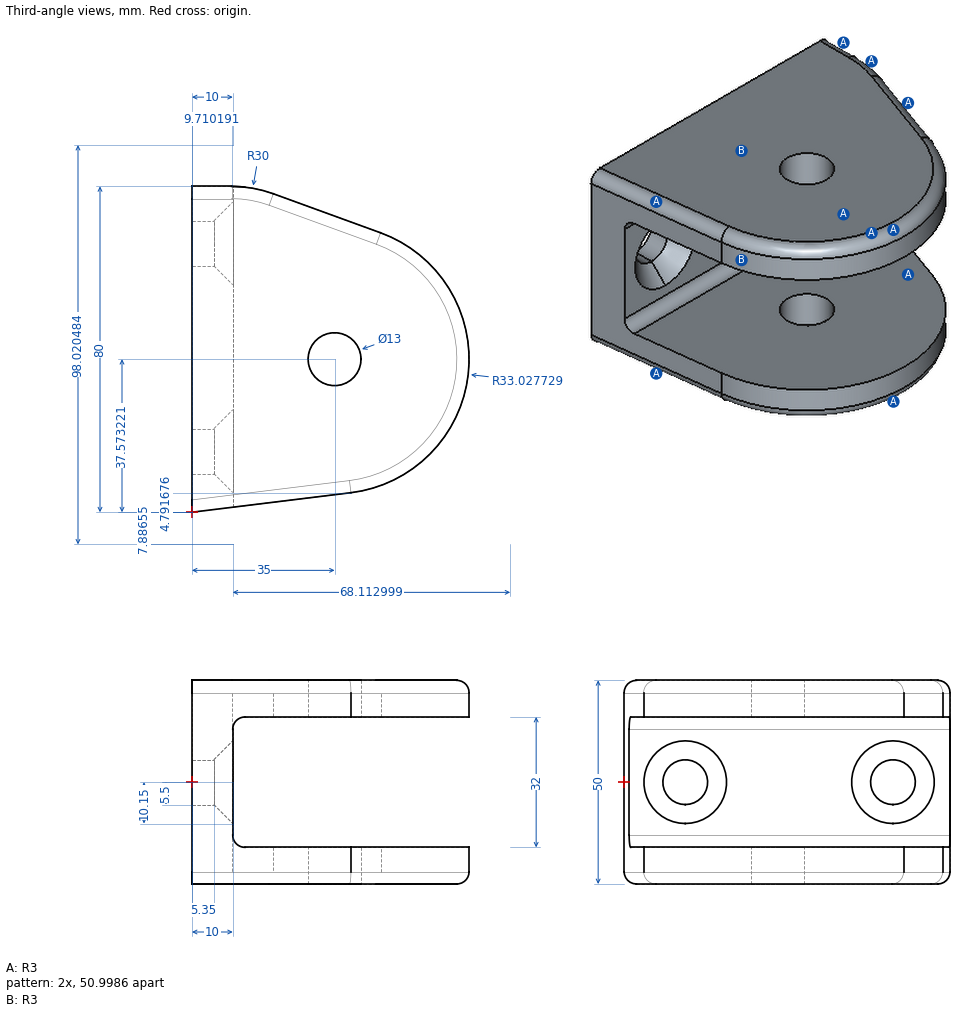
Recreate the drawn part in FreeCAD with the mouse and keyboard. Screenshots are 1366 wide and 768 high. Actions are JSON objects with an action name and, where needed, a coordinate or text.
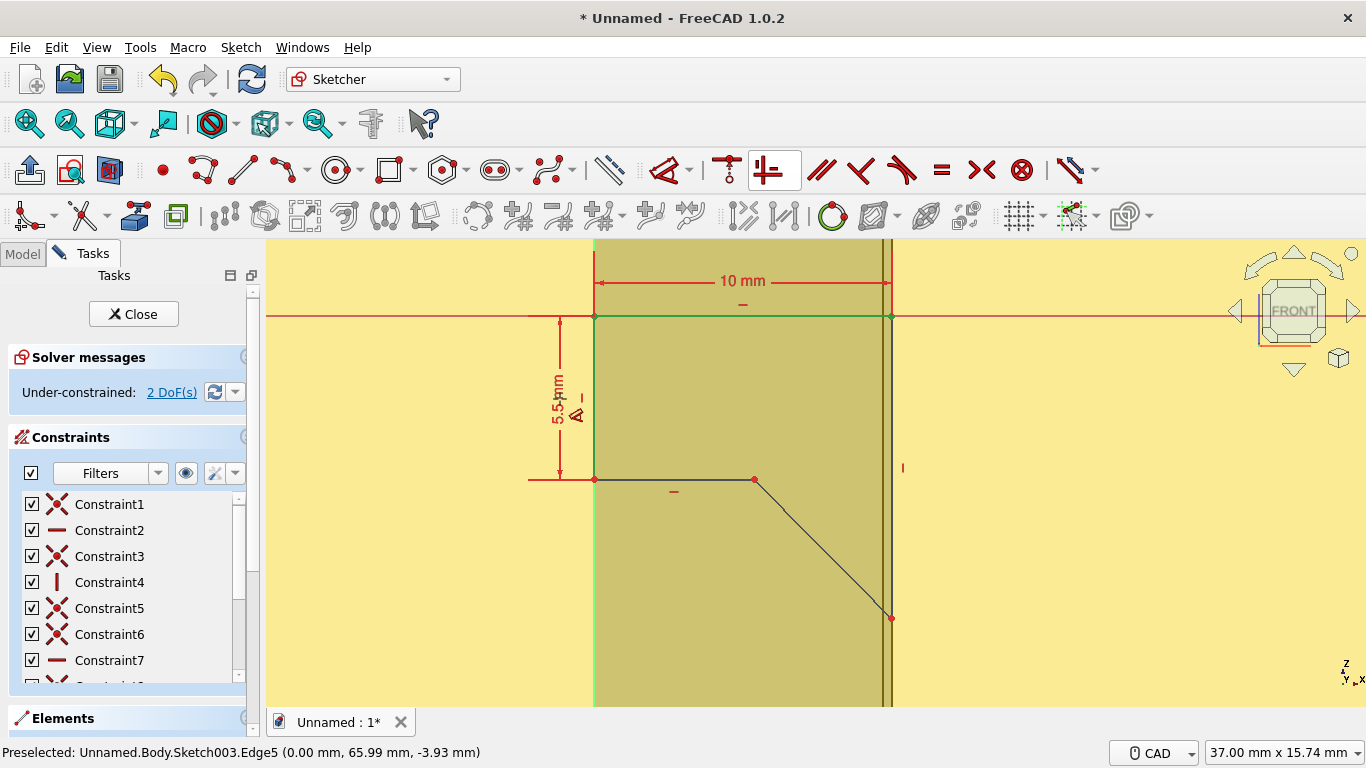
{"action": "left_click", "coordinate": [706, 480]}
{"action": "left_click", "coordinate": [674, 514]}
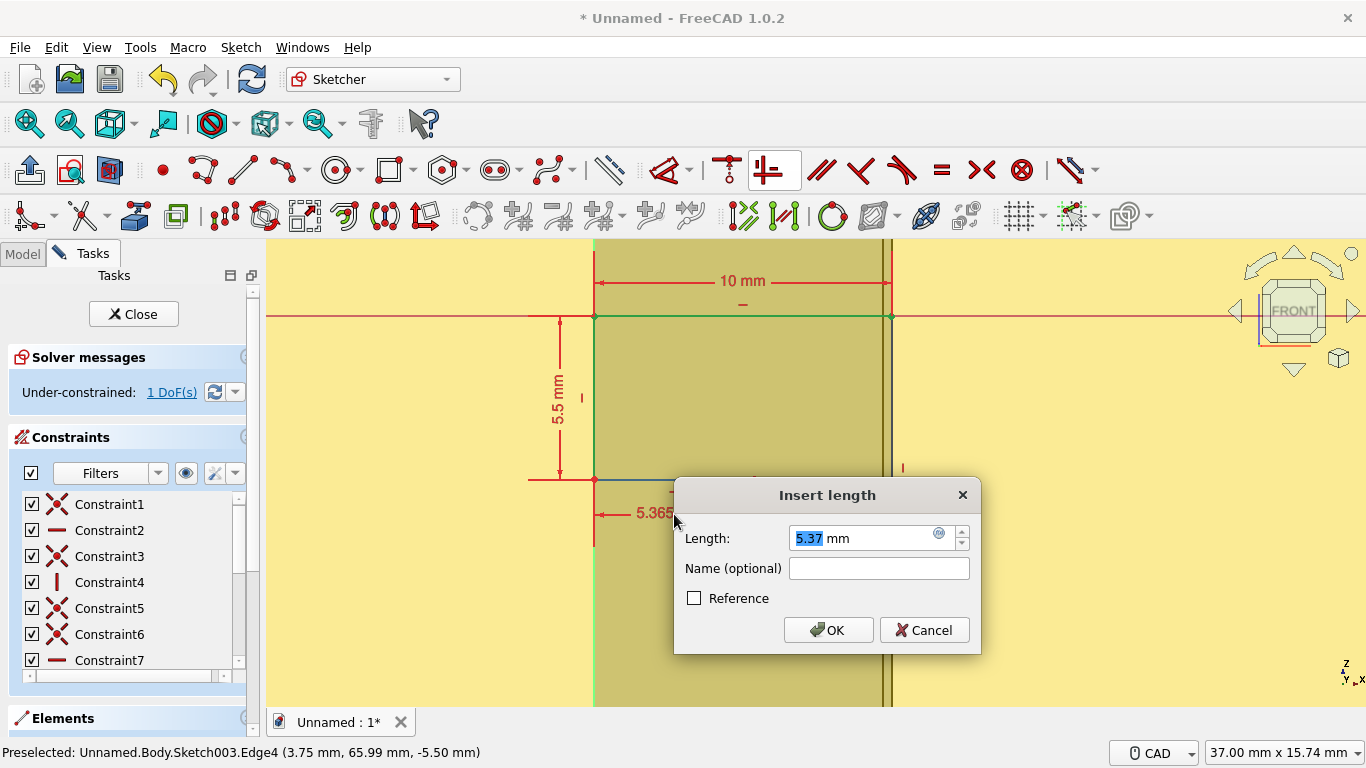
{"action": "type", "text": "5.35"}
{"action": "key", "text": "Return"}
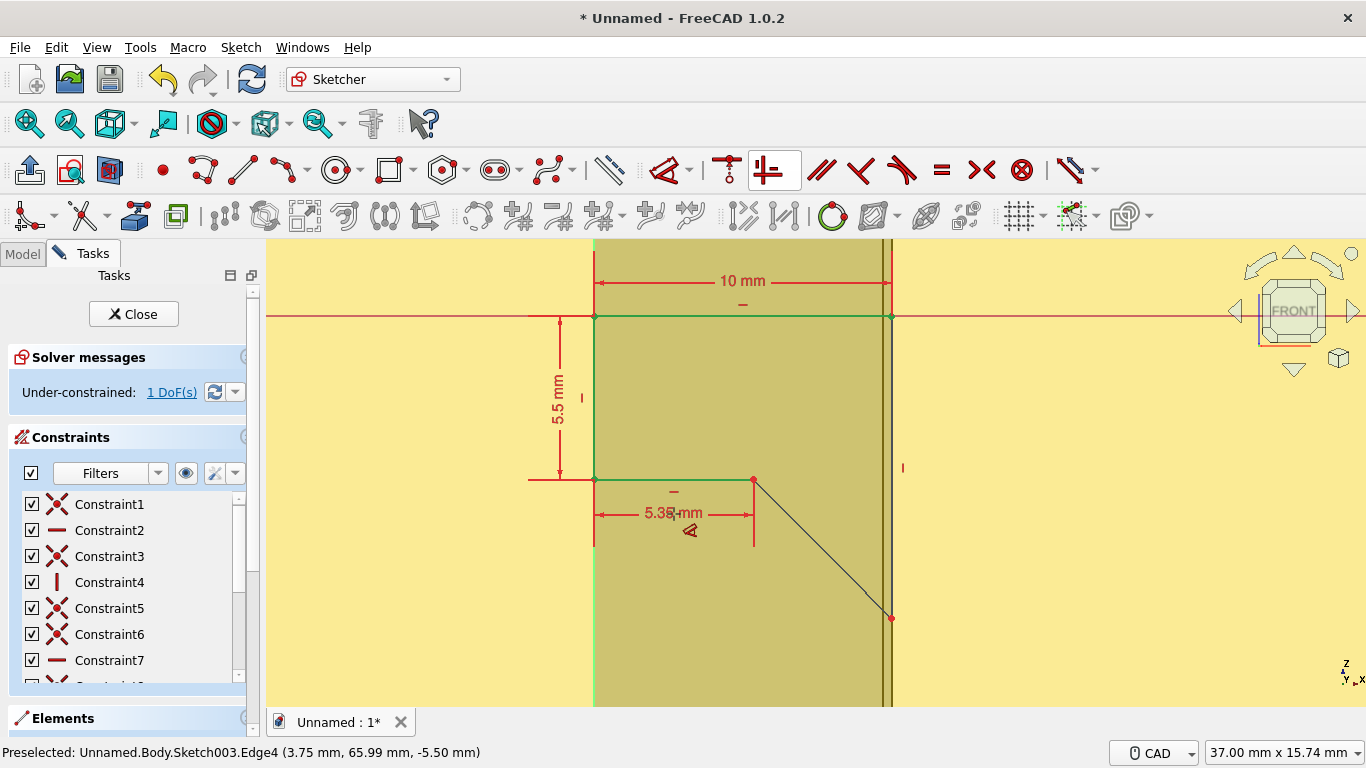
{"action": "left_click", "coordinate": [892, 407]}
{"action": "left_click", "coordinate": [926, 468]}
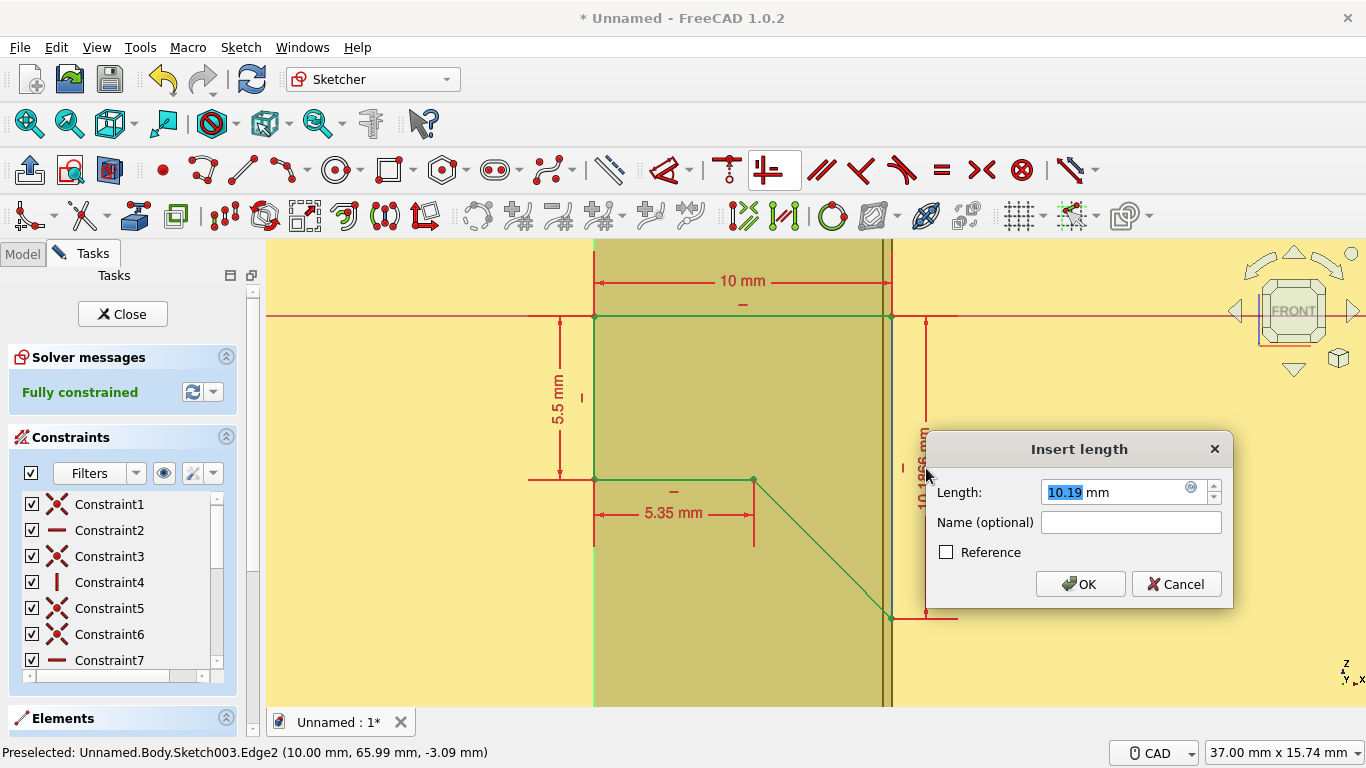
{"action": "type", "text": "10.15"}
{"action": "key", "text": "Return"}
{"action": "key", "text": "Escape"}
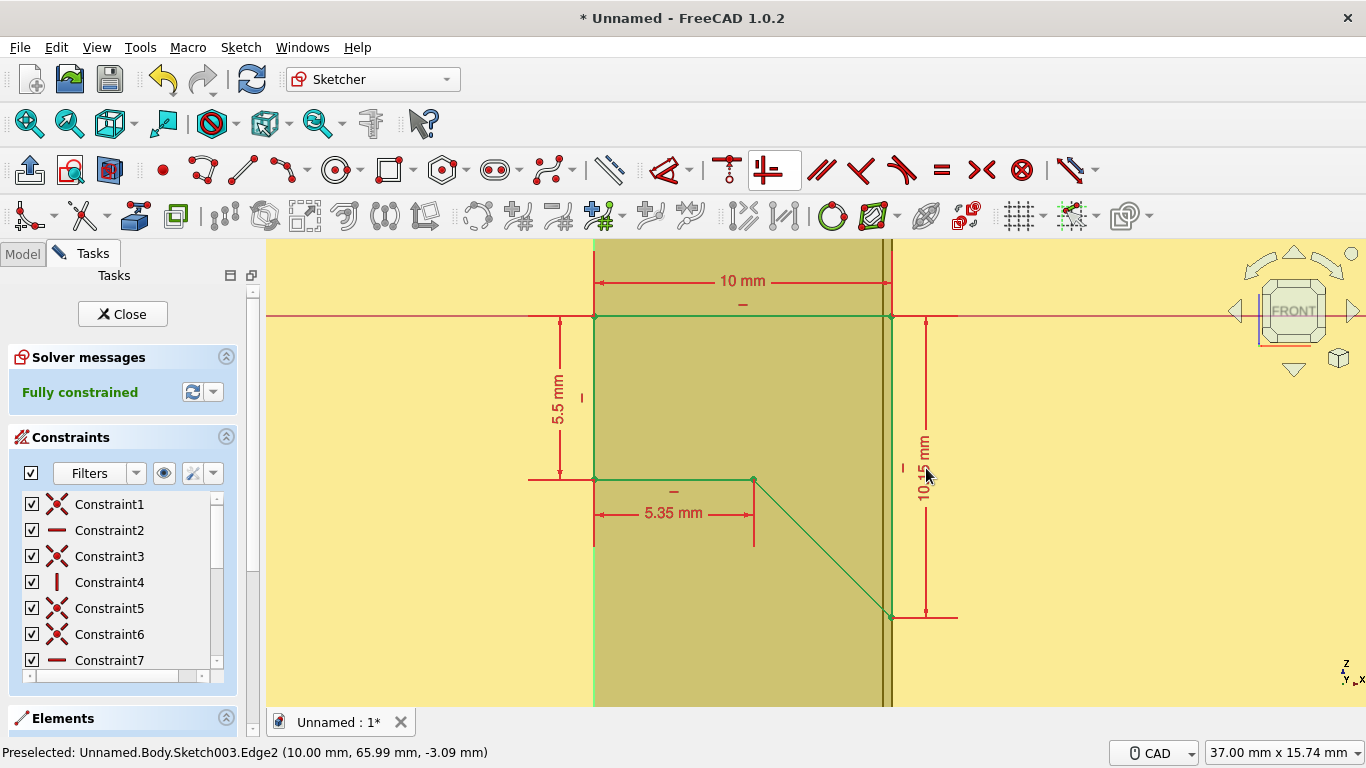
{"action": "left_click", "coordinate": [123, 314]}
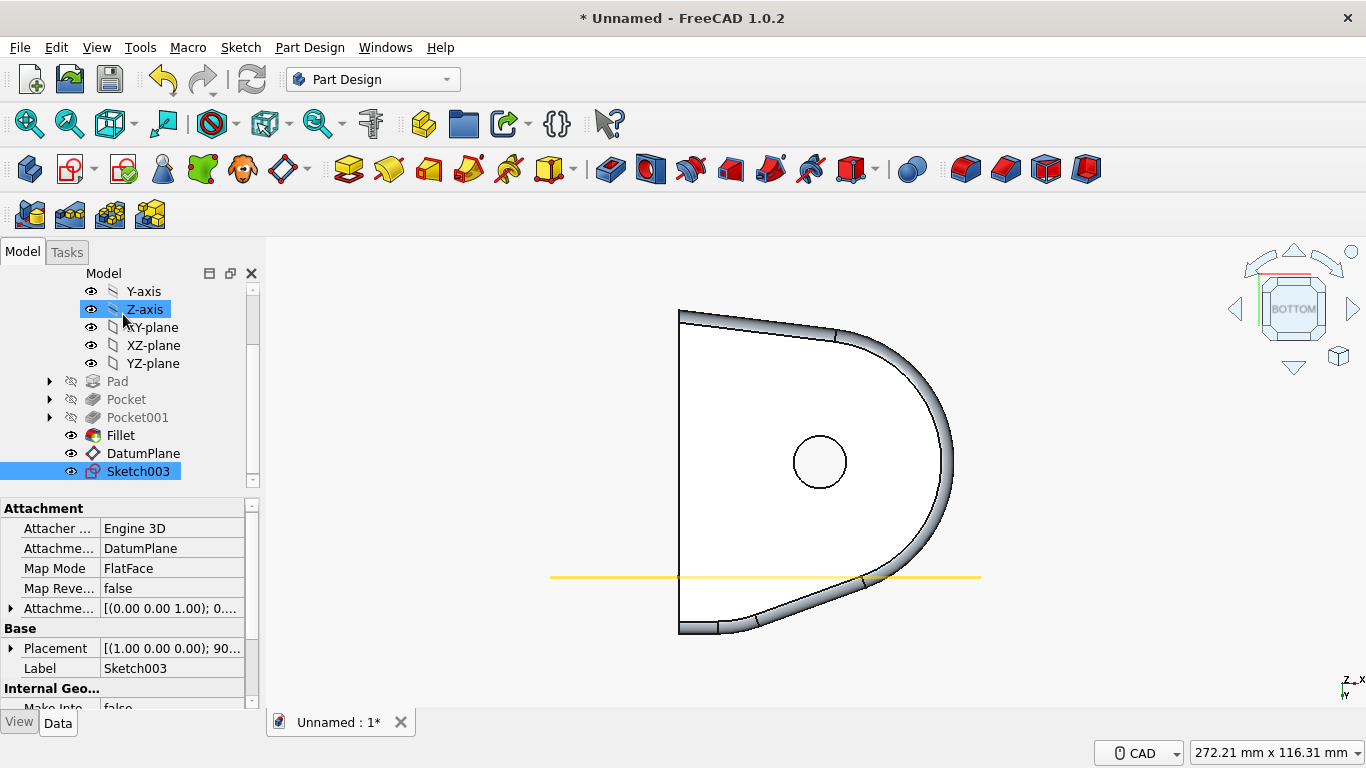
{"action": "left_click", "coordinate": [692, 170]}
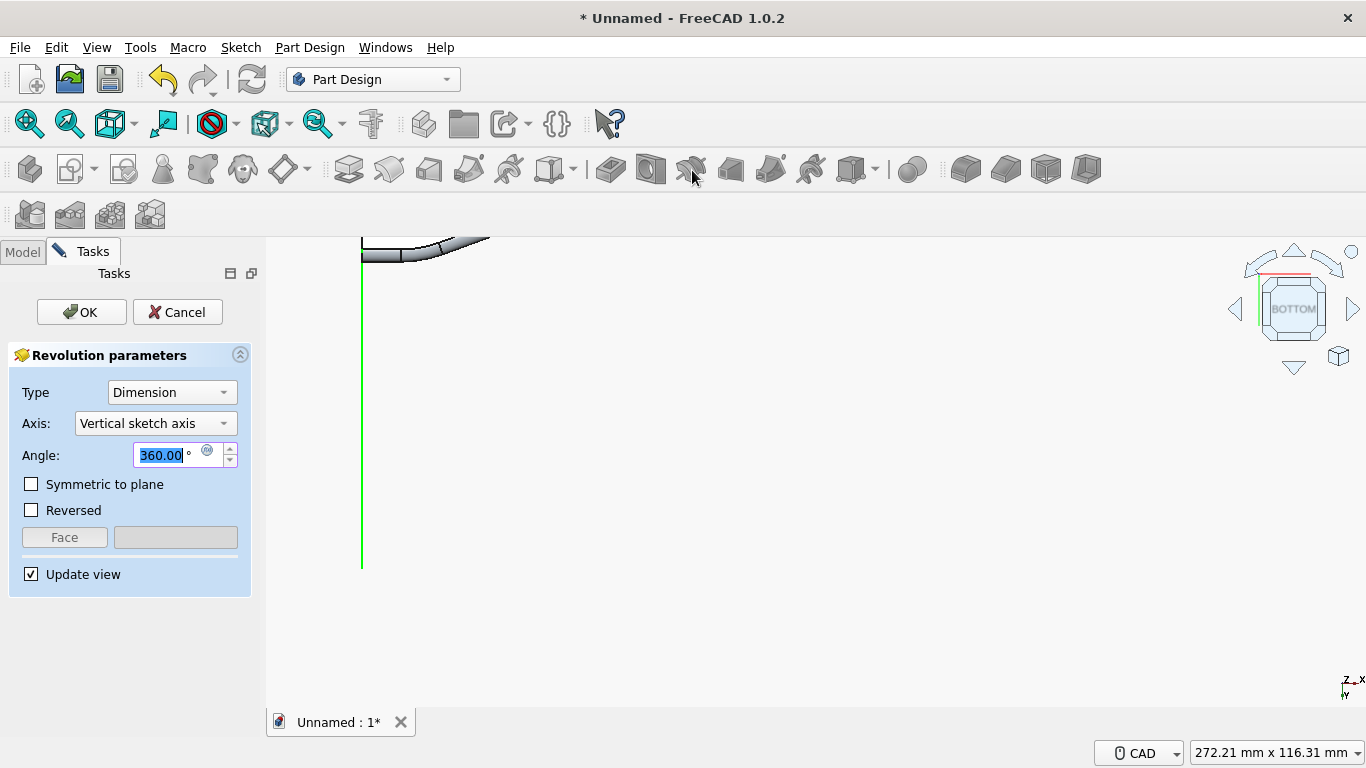
{"action": "left_click", "coordinate": [156, 424]}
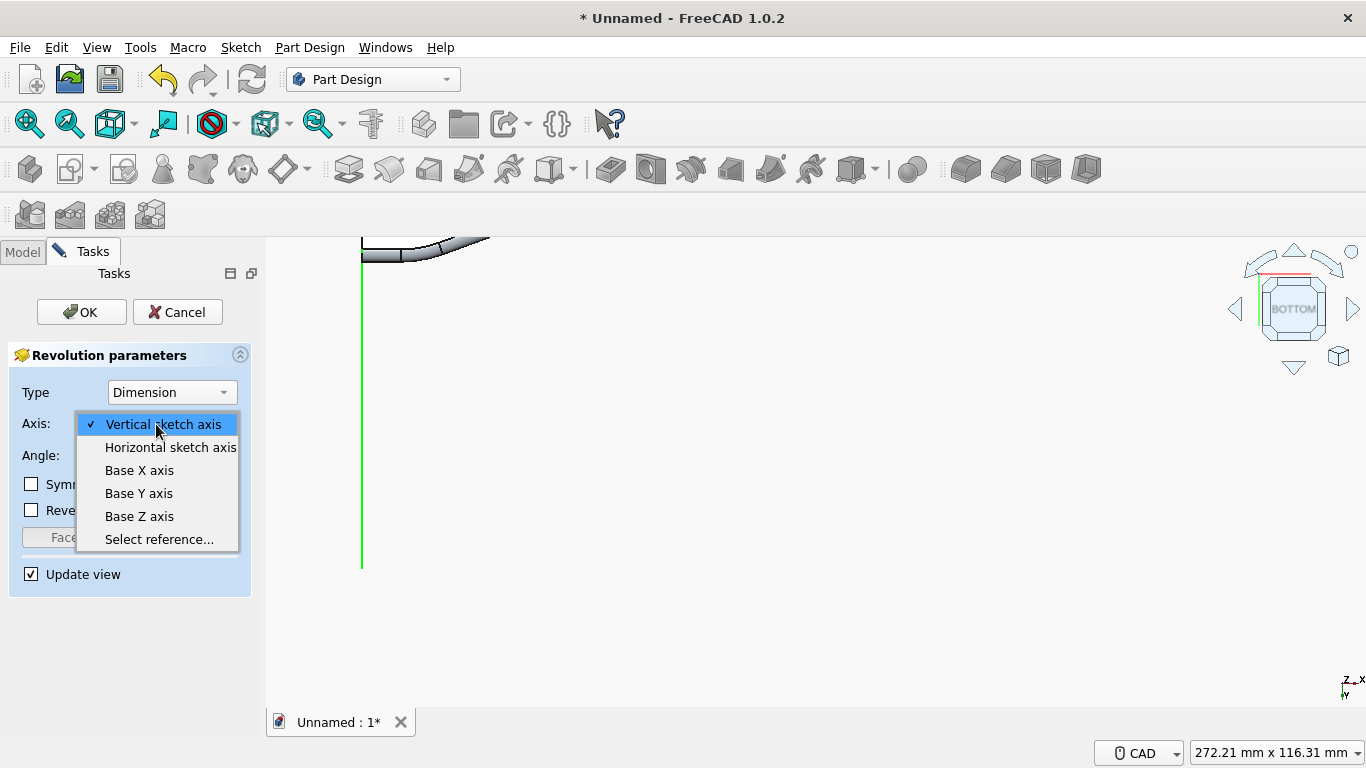
{"action": "left_click", "coordinate": [156, 448]}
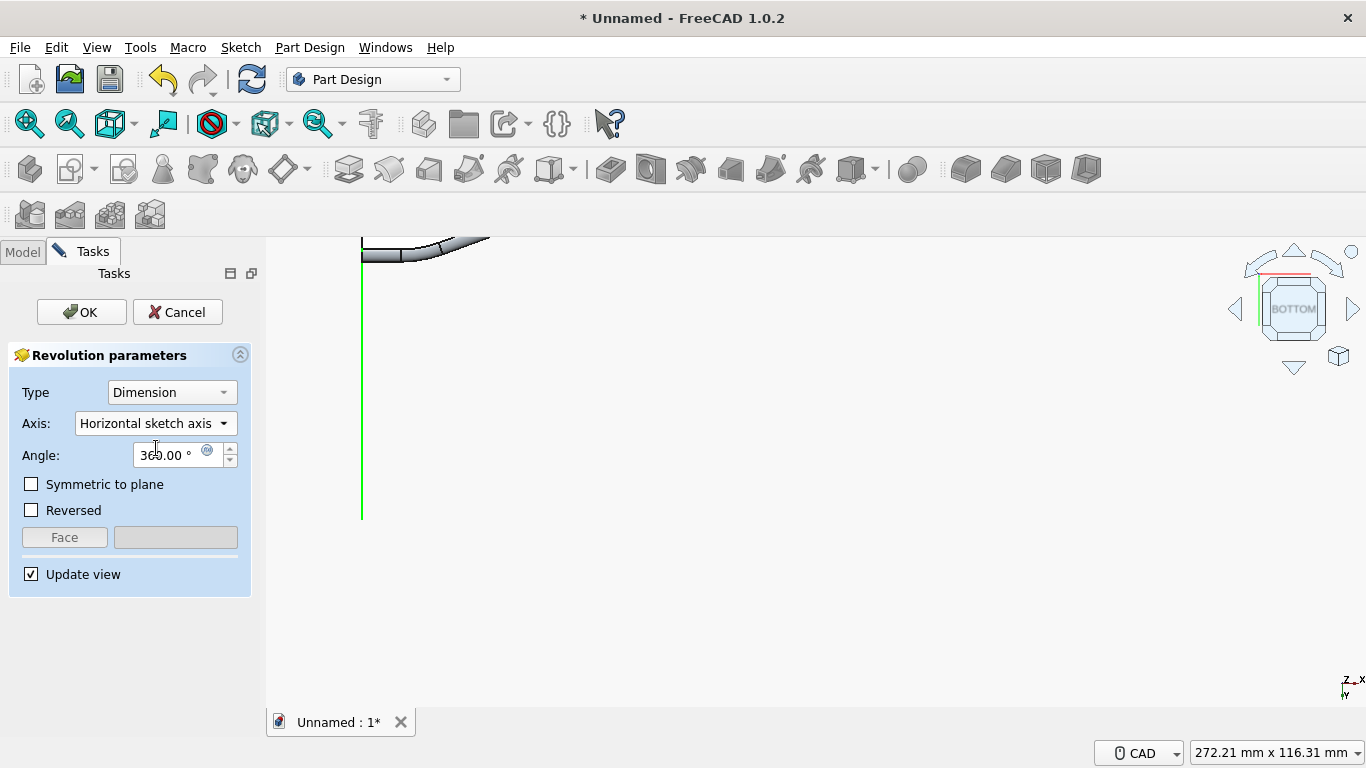
{"action": "left_click", "coordinate": [82, 312]}